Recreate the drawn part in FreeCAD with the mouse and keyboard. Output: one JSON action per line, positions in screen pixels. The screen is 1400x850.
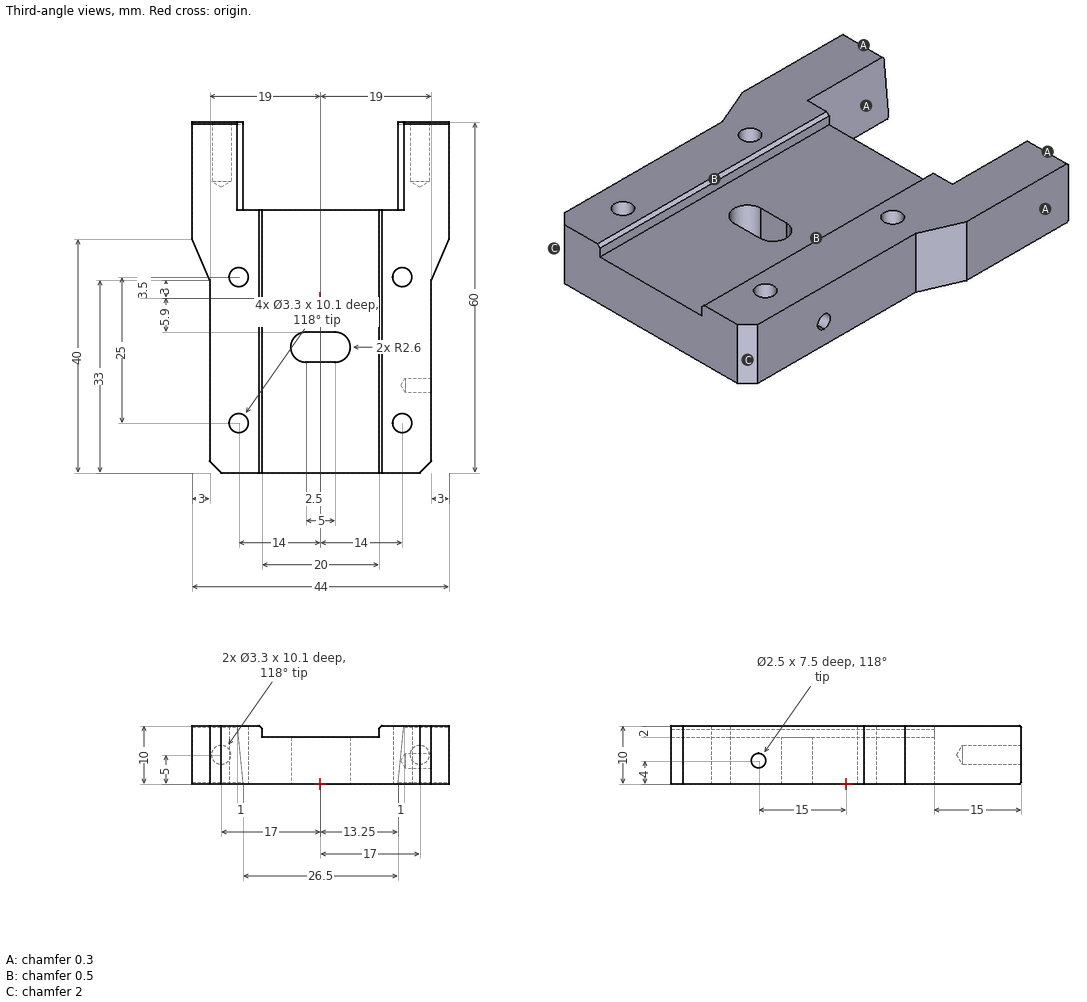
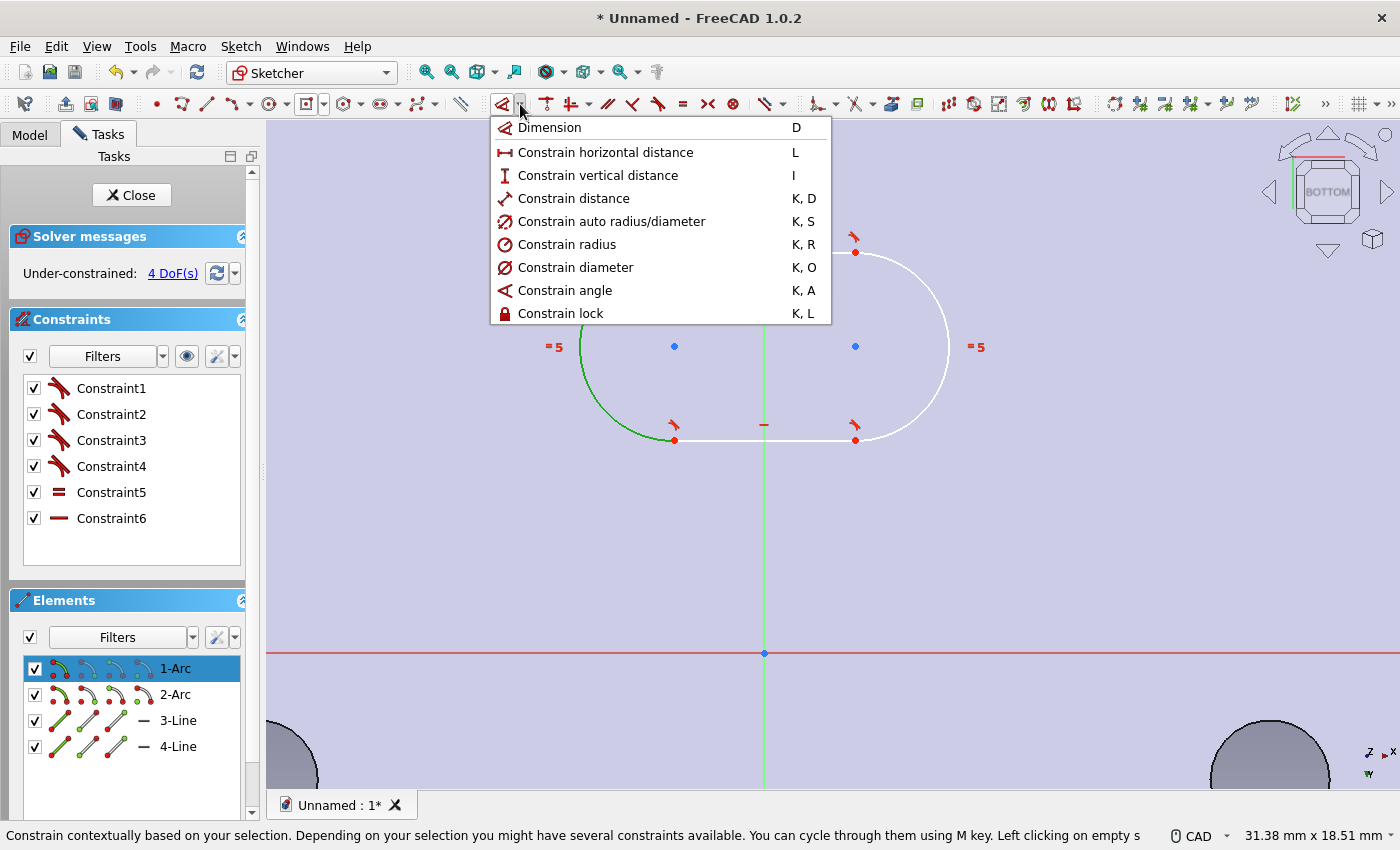
{"action": "left_click", "coordinate": [661, 244]}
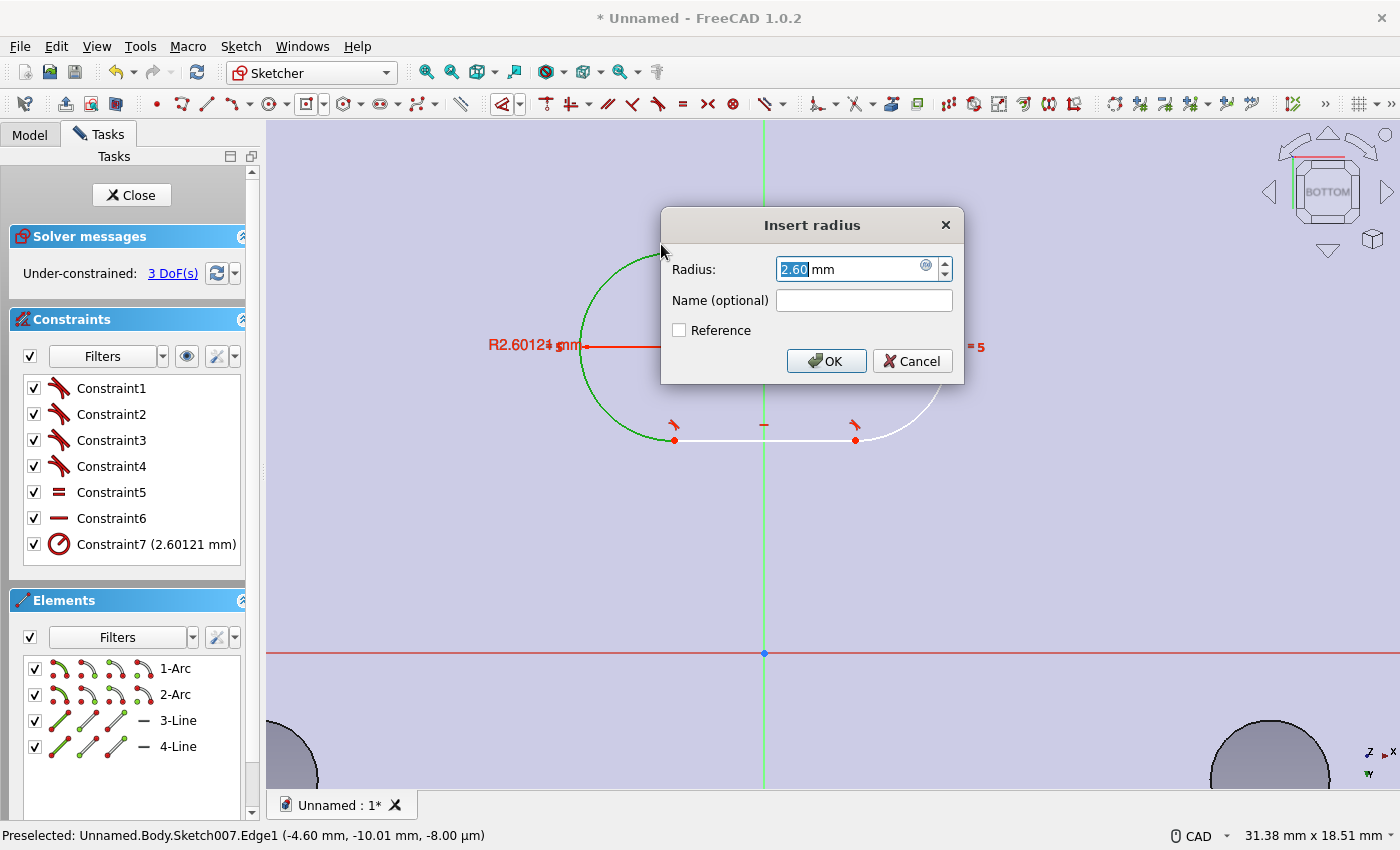
{"action": "type", "text": "2.6"}
{"action": "key", "text": "Return"}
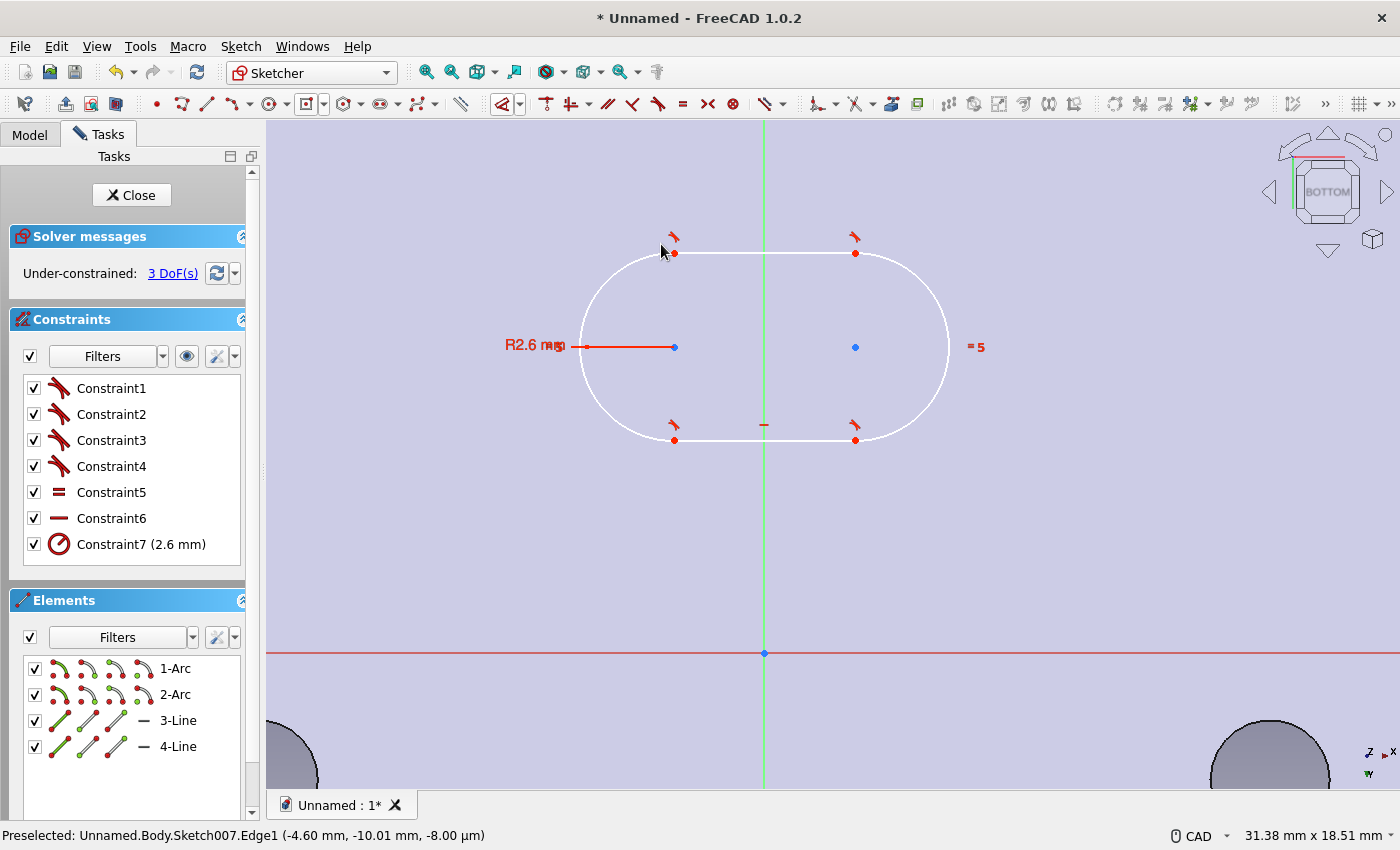
{"action": "left_click", "coordinate": [728, 253]}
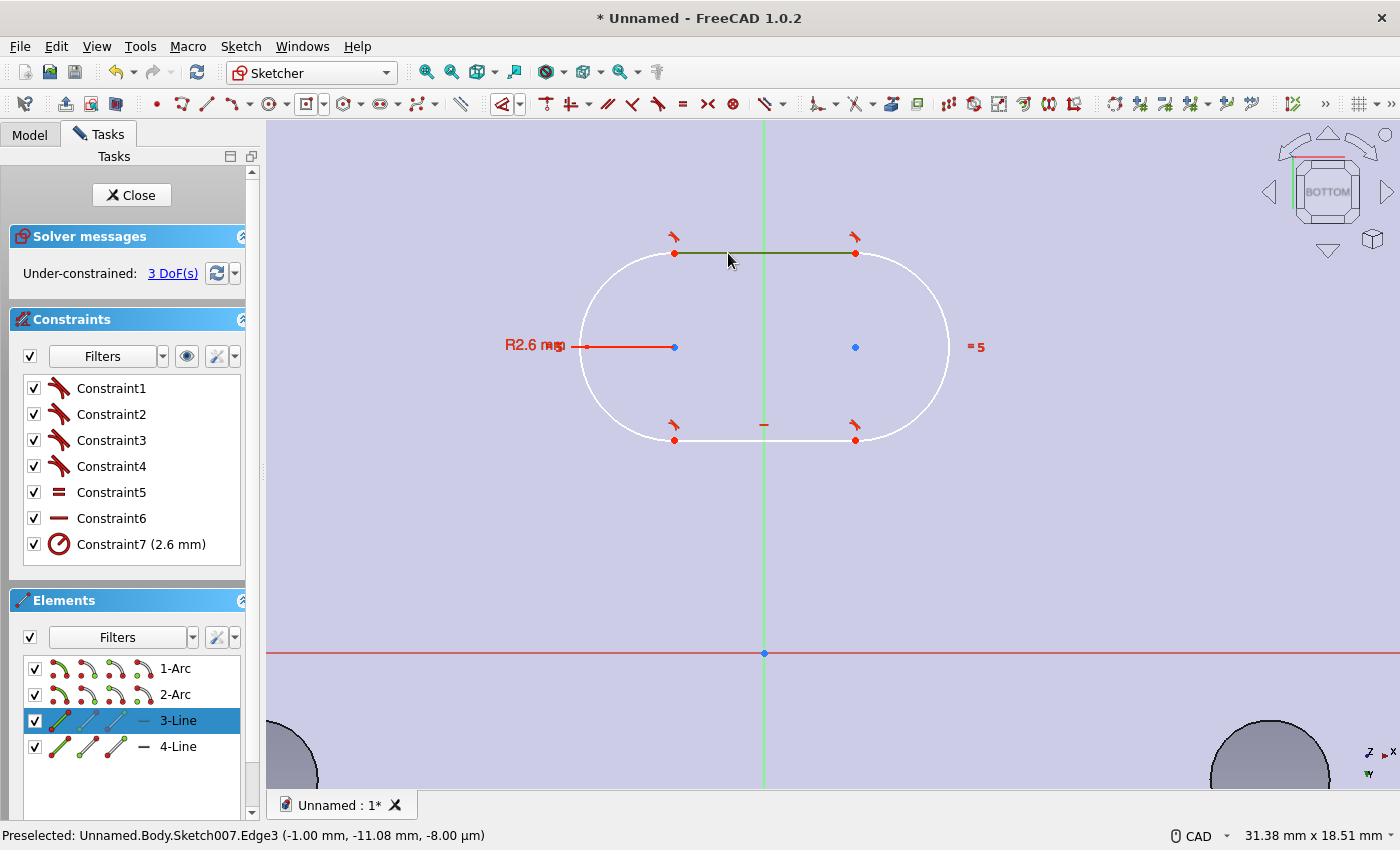
{"action": "key", "text": "l"}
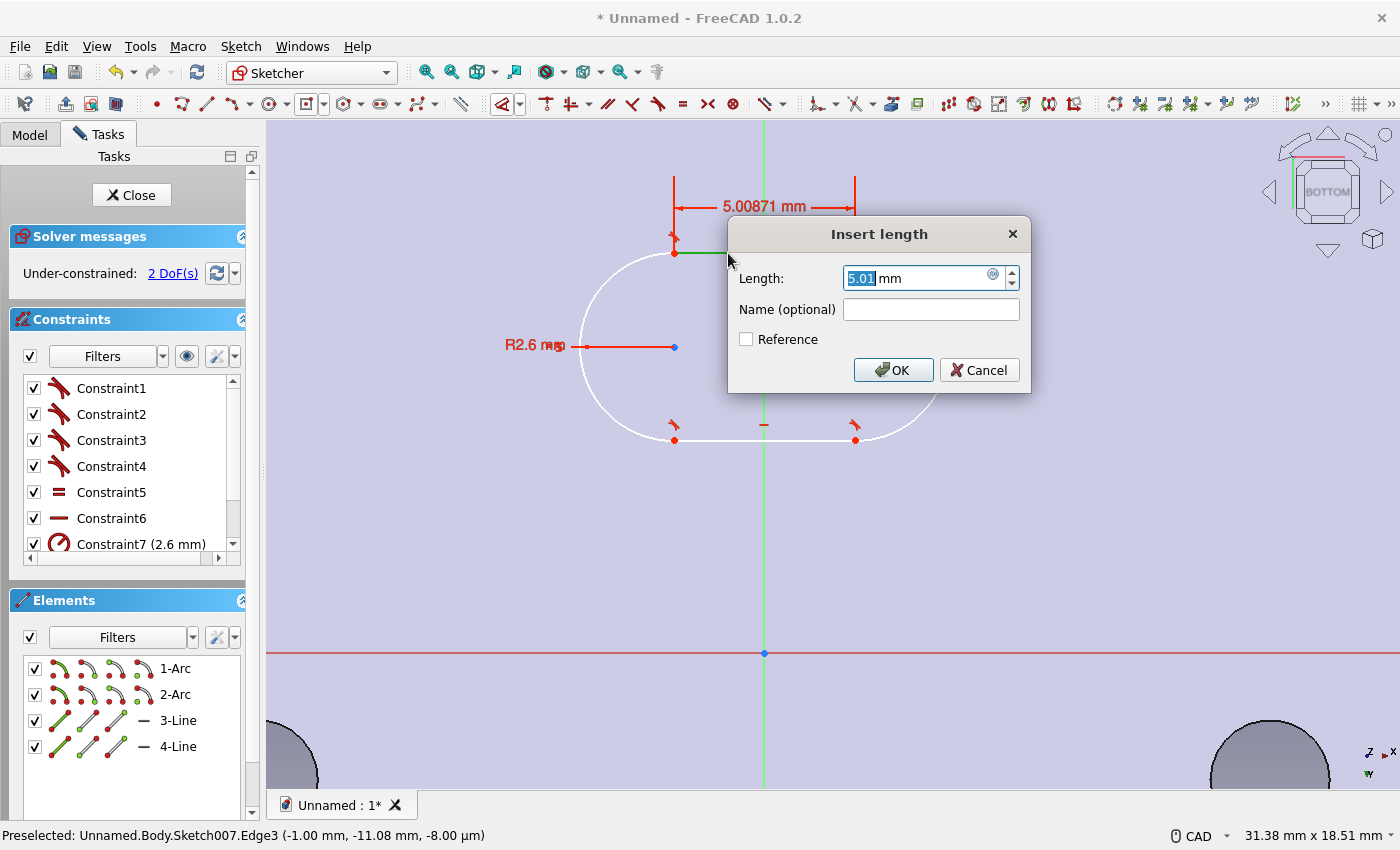
{"action": "type", "text": "5"}
{"action": "key", "text": "Return"}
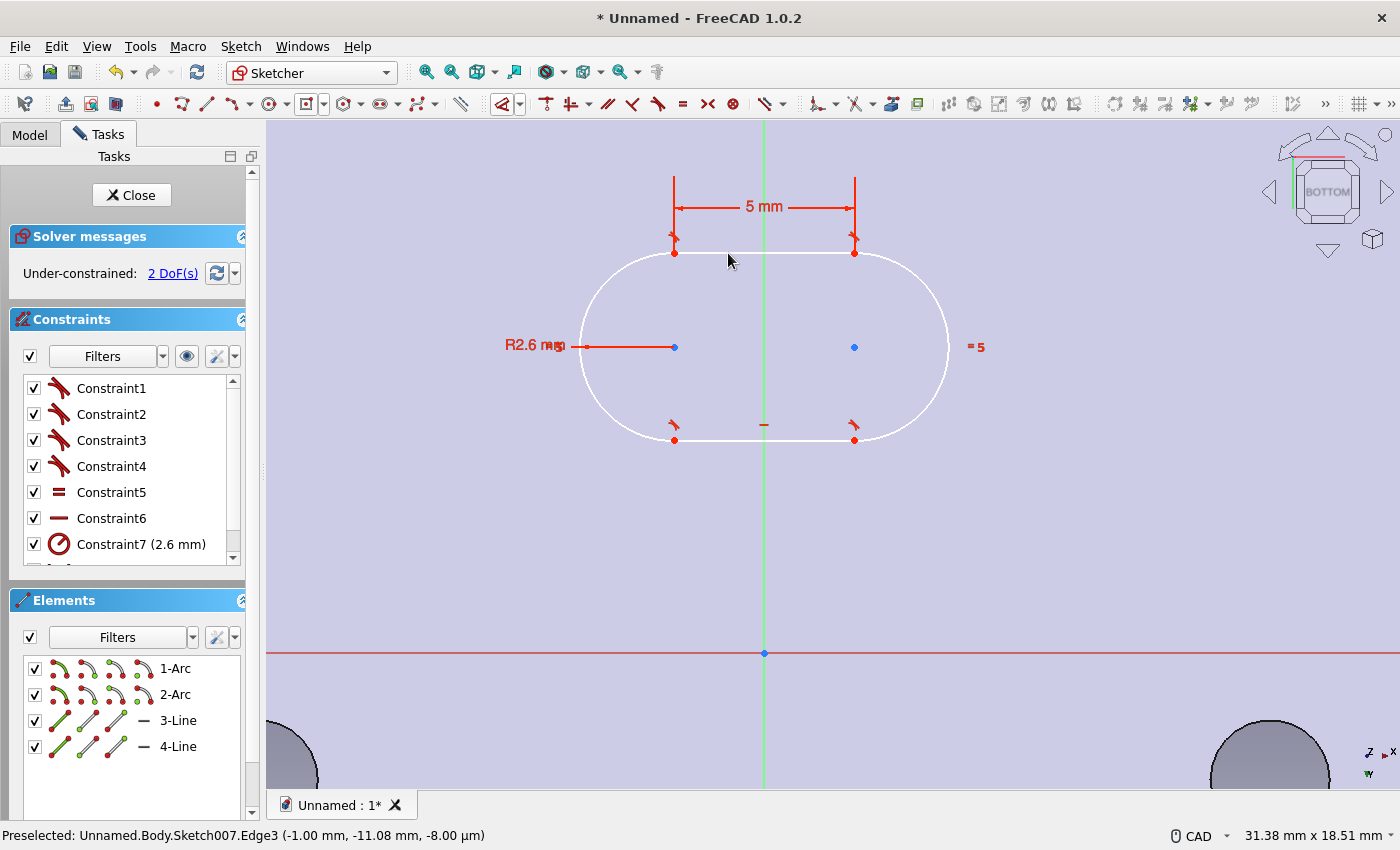
{"action": "left_click", "coordinate": [674, 253]}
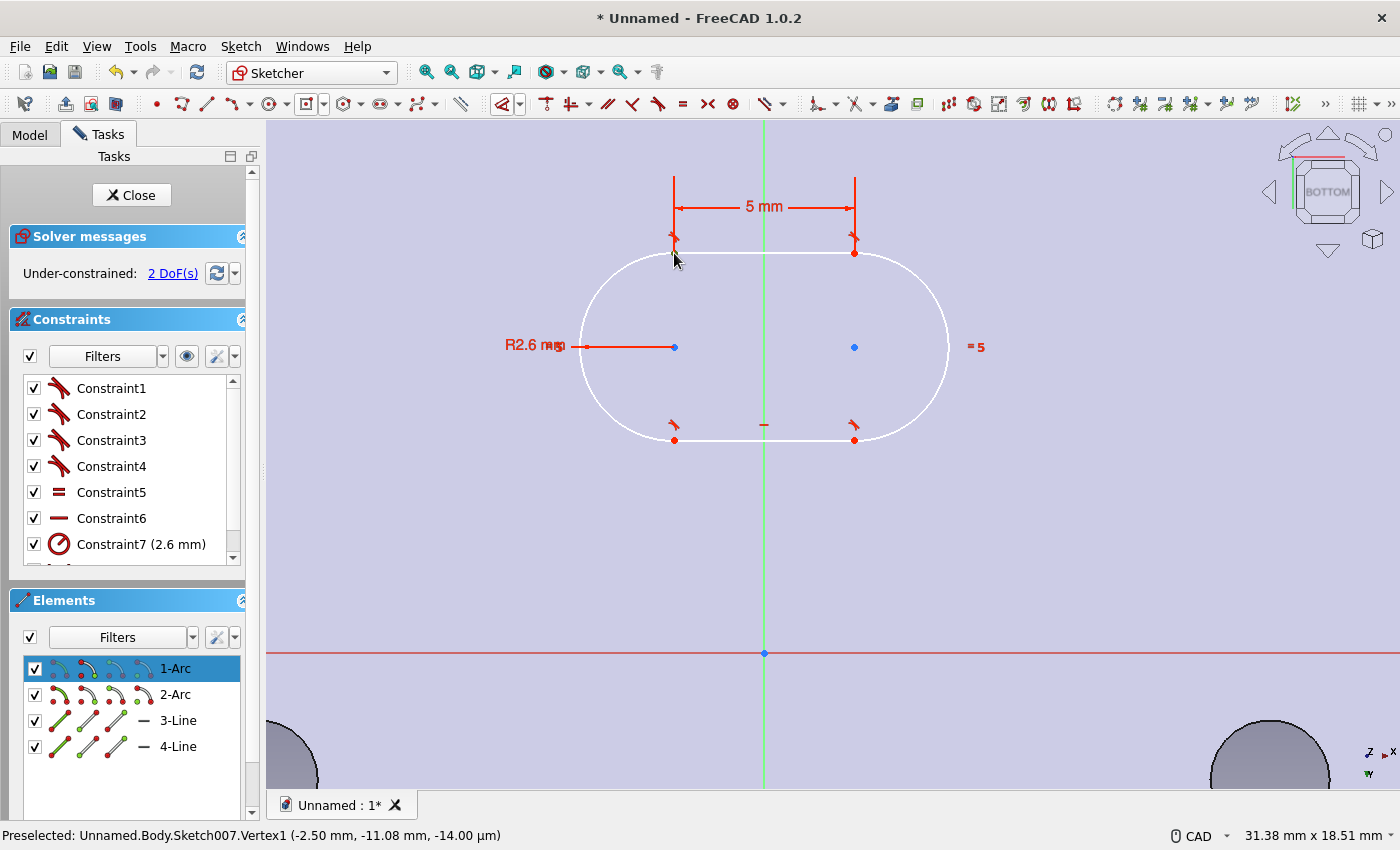
{"action": "key", "text": "l"}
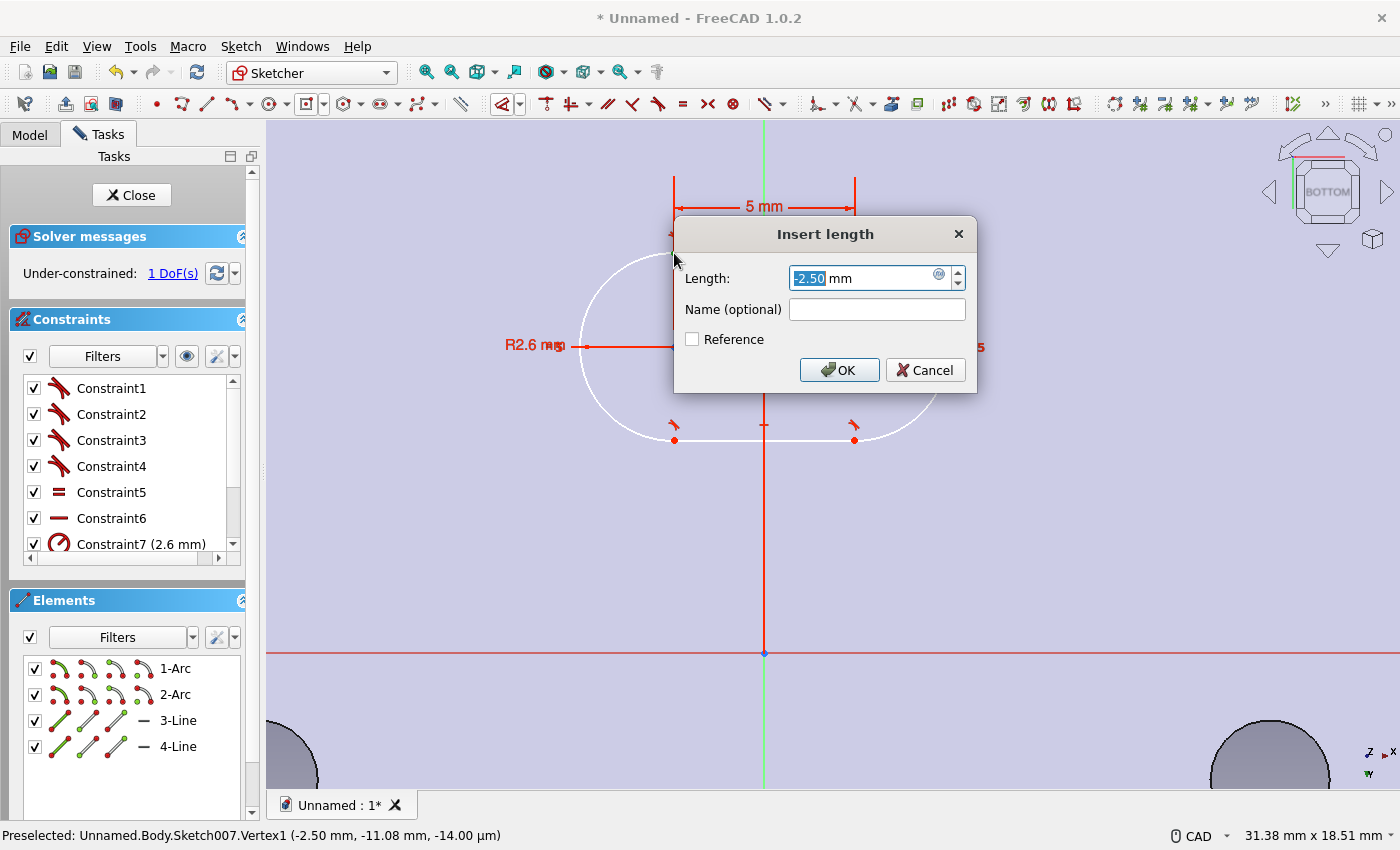
{"action": "type", "text": "-2.5"}
{"action": "key", "text": "Return"}